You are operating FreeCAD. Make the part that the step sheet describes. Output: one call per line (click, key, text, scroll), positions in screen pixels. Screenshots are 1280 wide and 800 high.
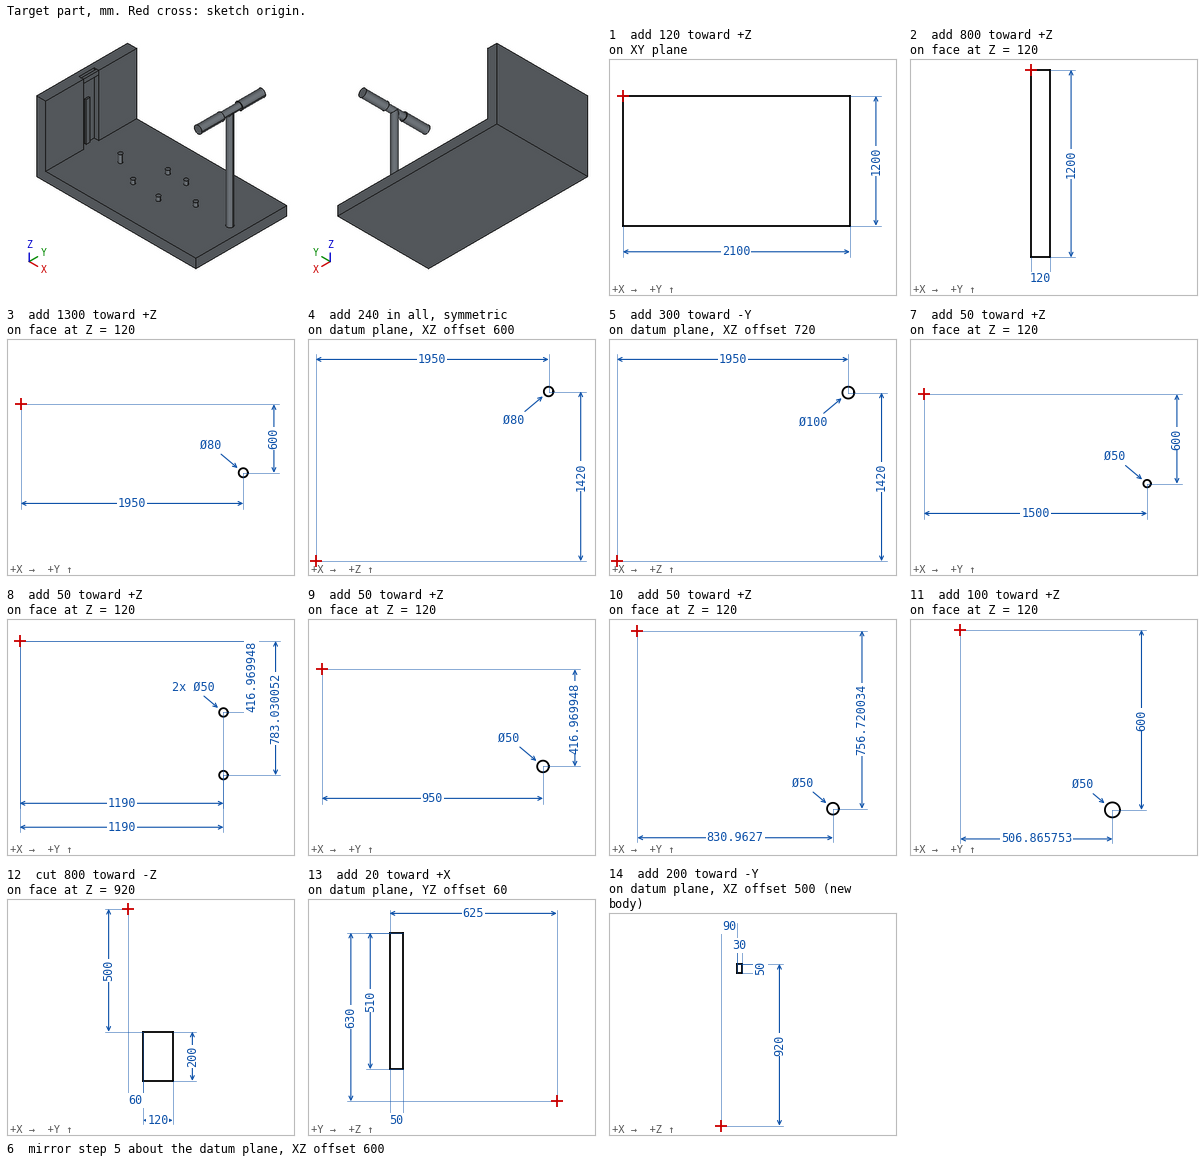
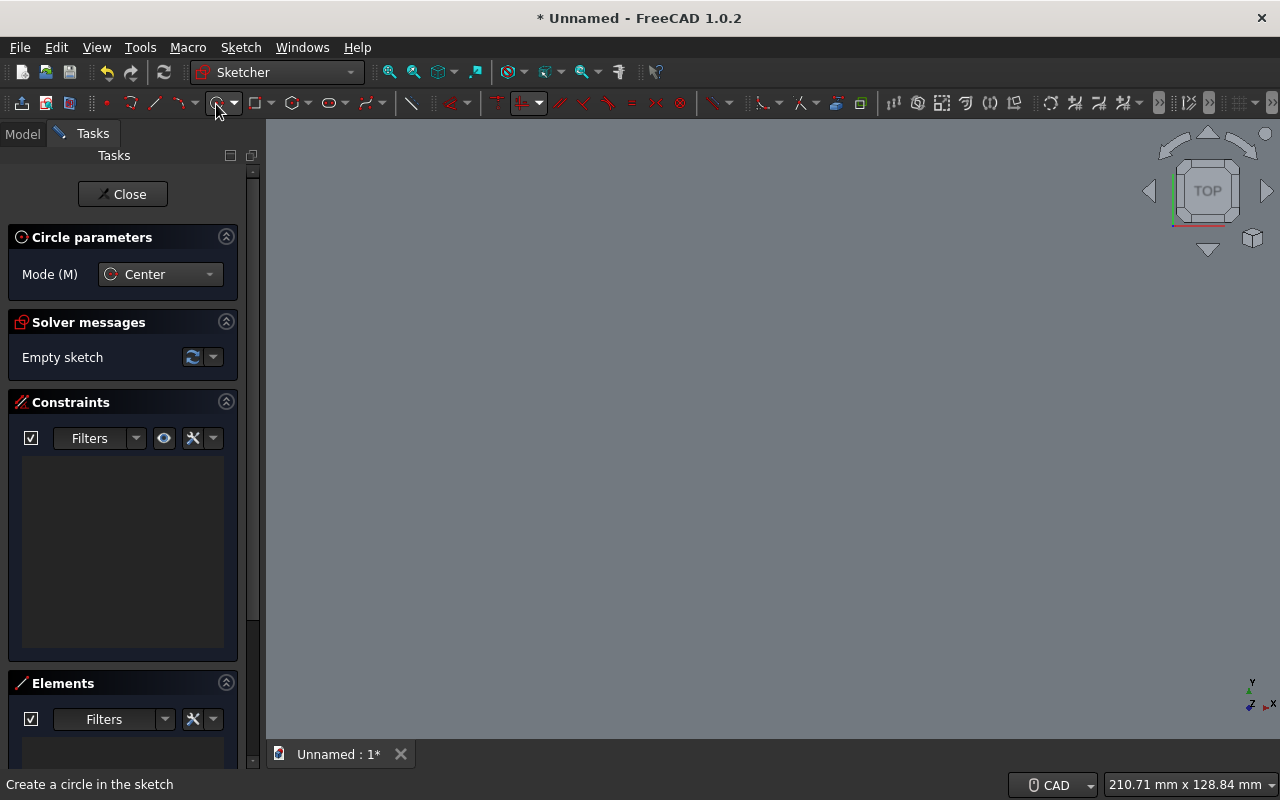
click(681, 419)
move(818, 283)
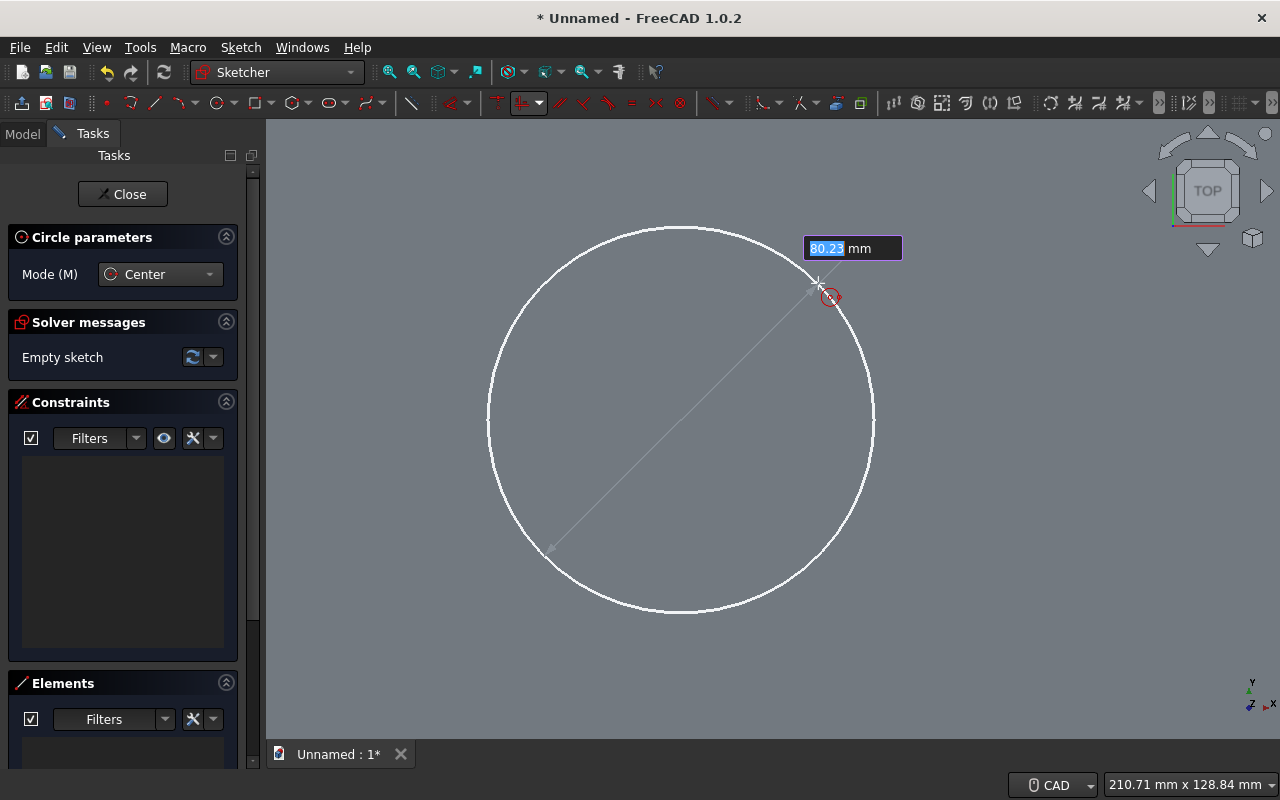
text(80)
key(Return)
key(Escape)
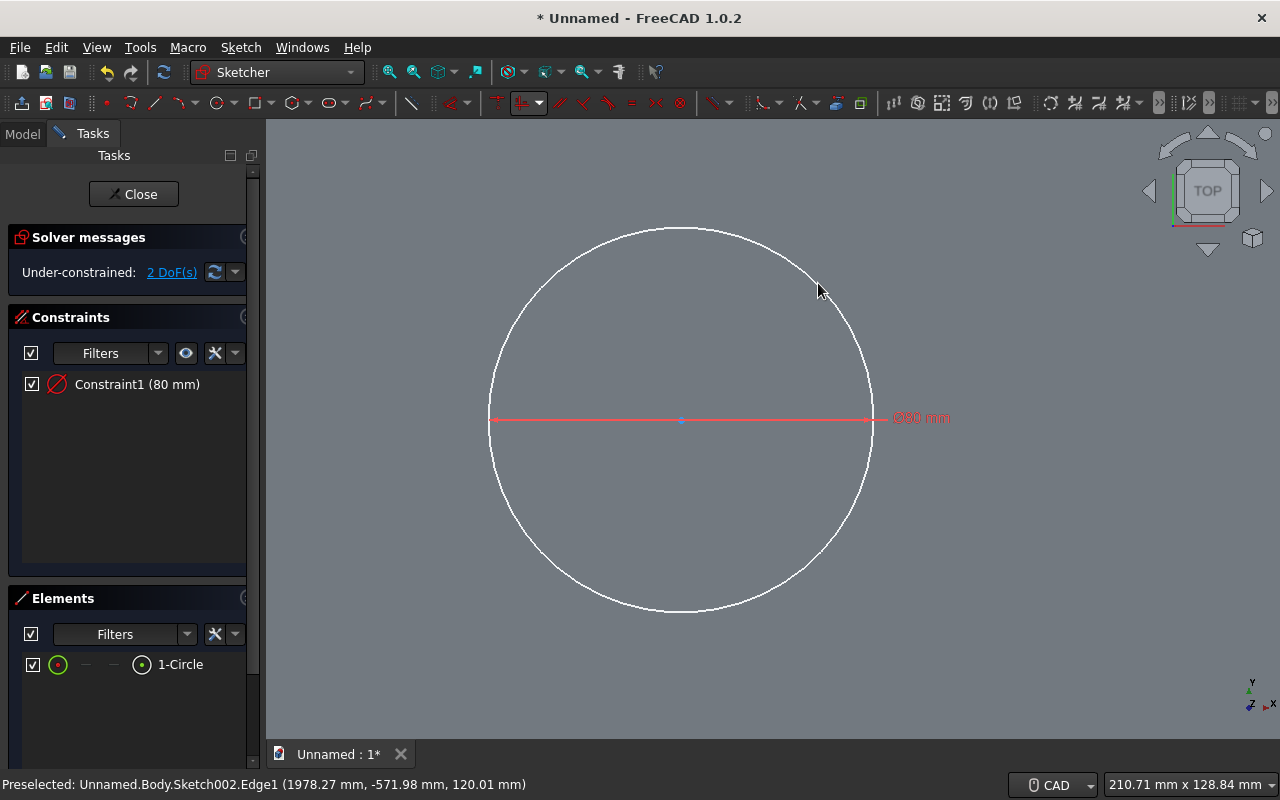
click(450, 104)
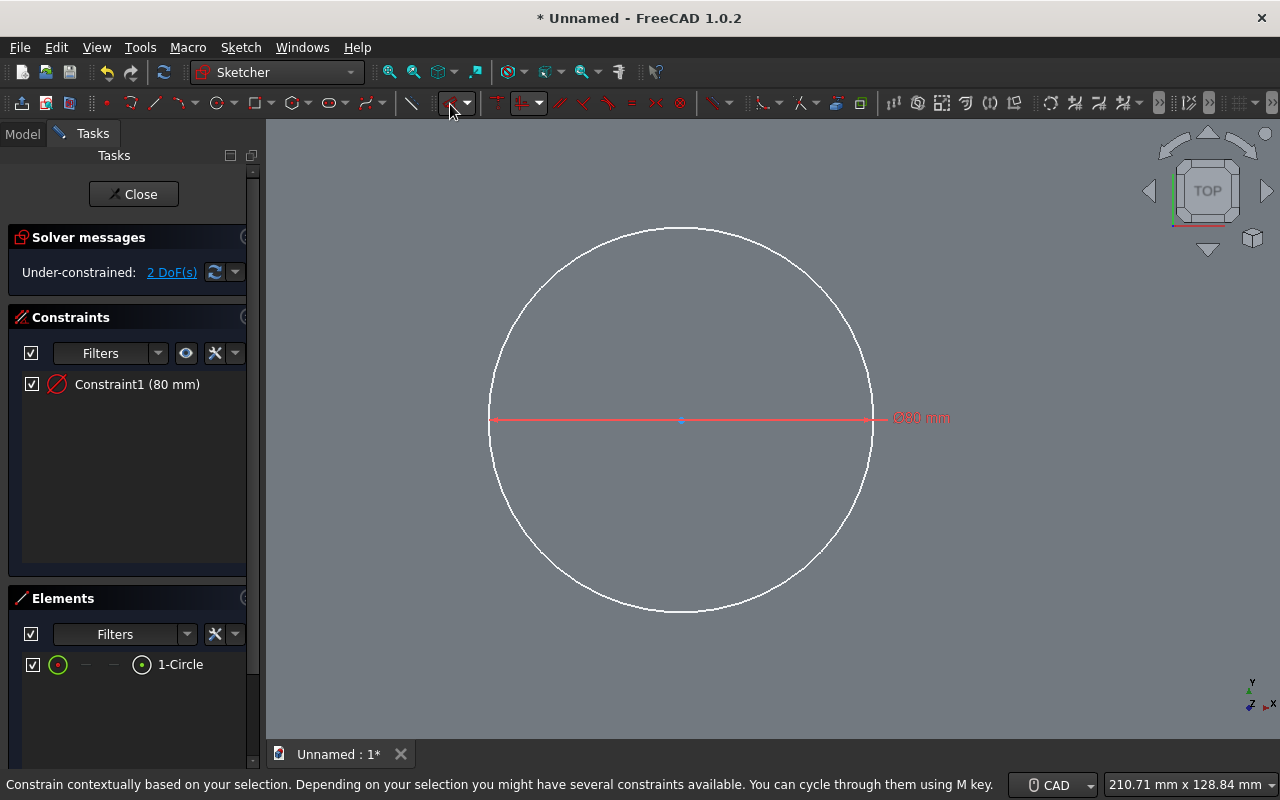
click(681, 420)
click(715, 284)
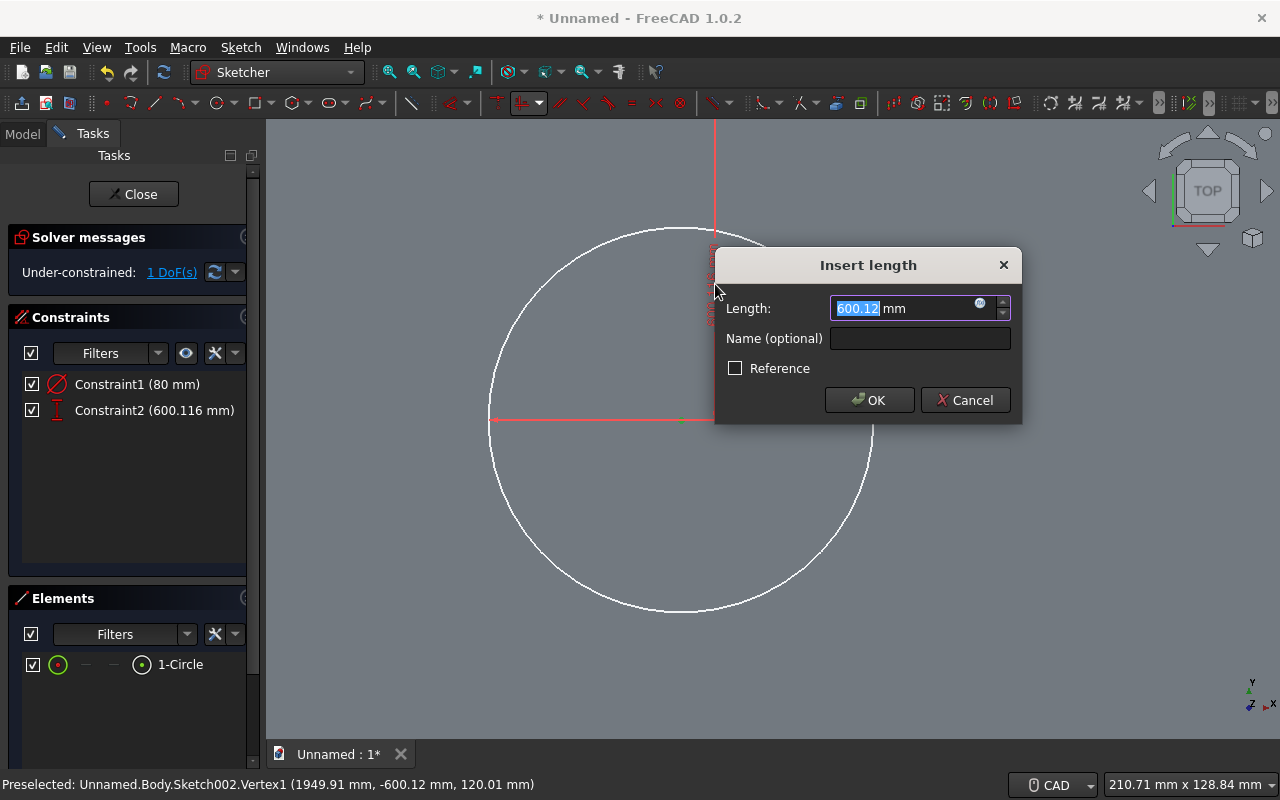
text(600)
key(Return)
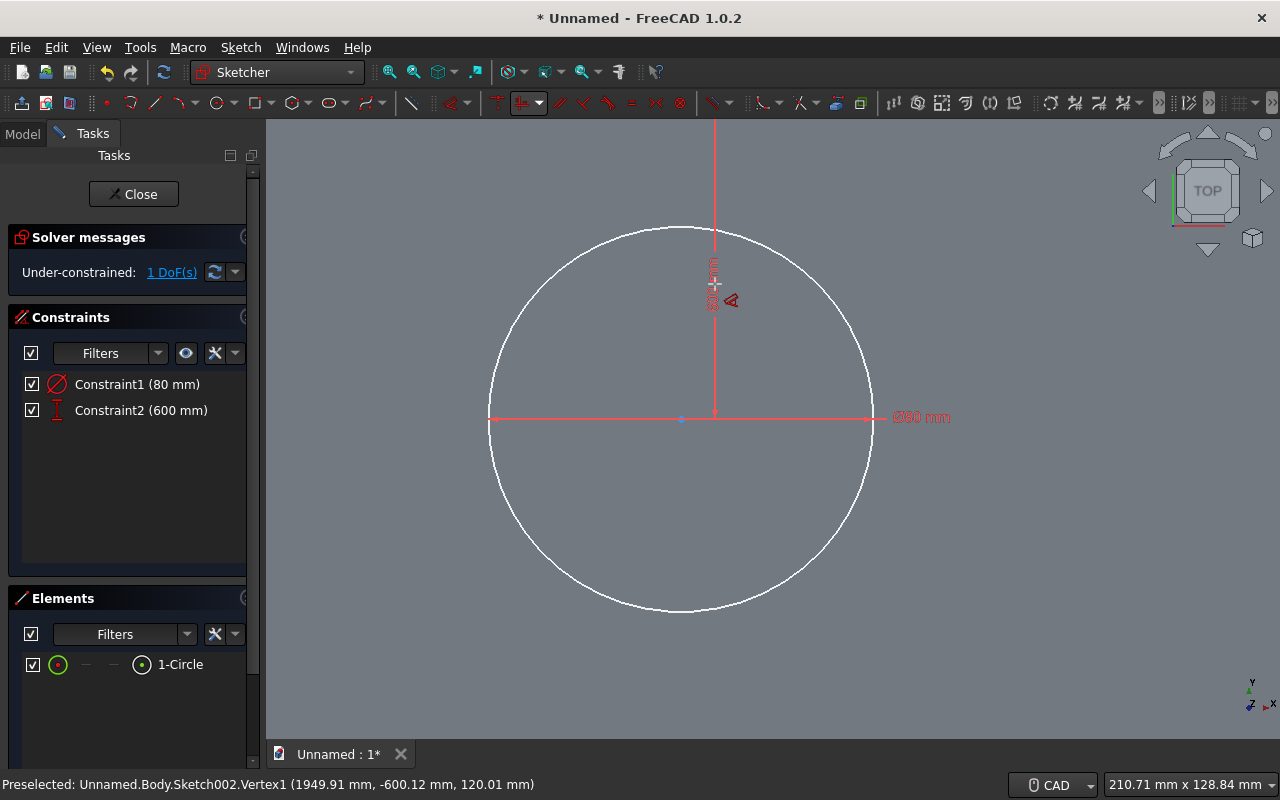
click(681, 419)
click(398, 453)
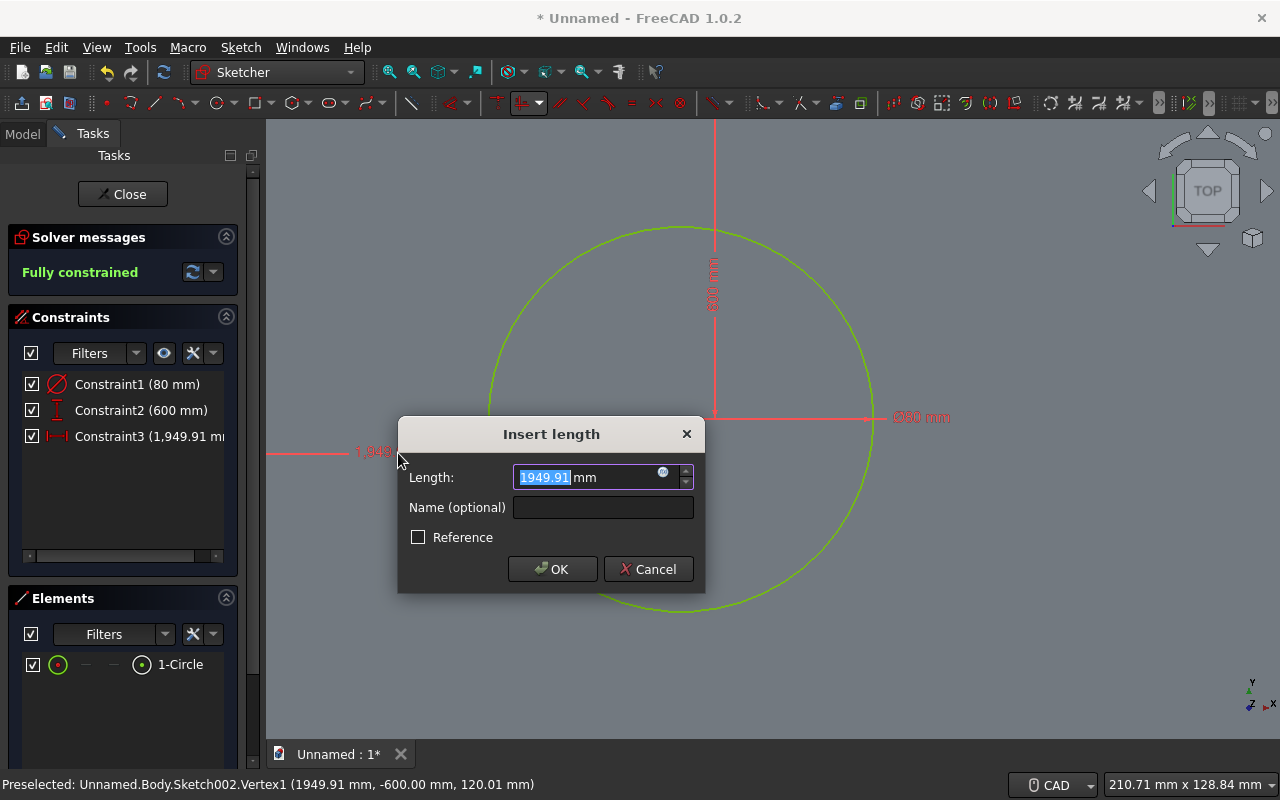
text(1950)
key(Return)
key(Escape)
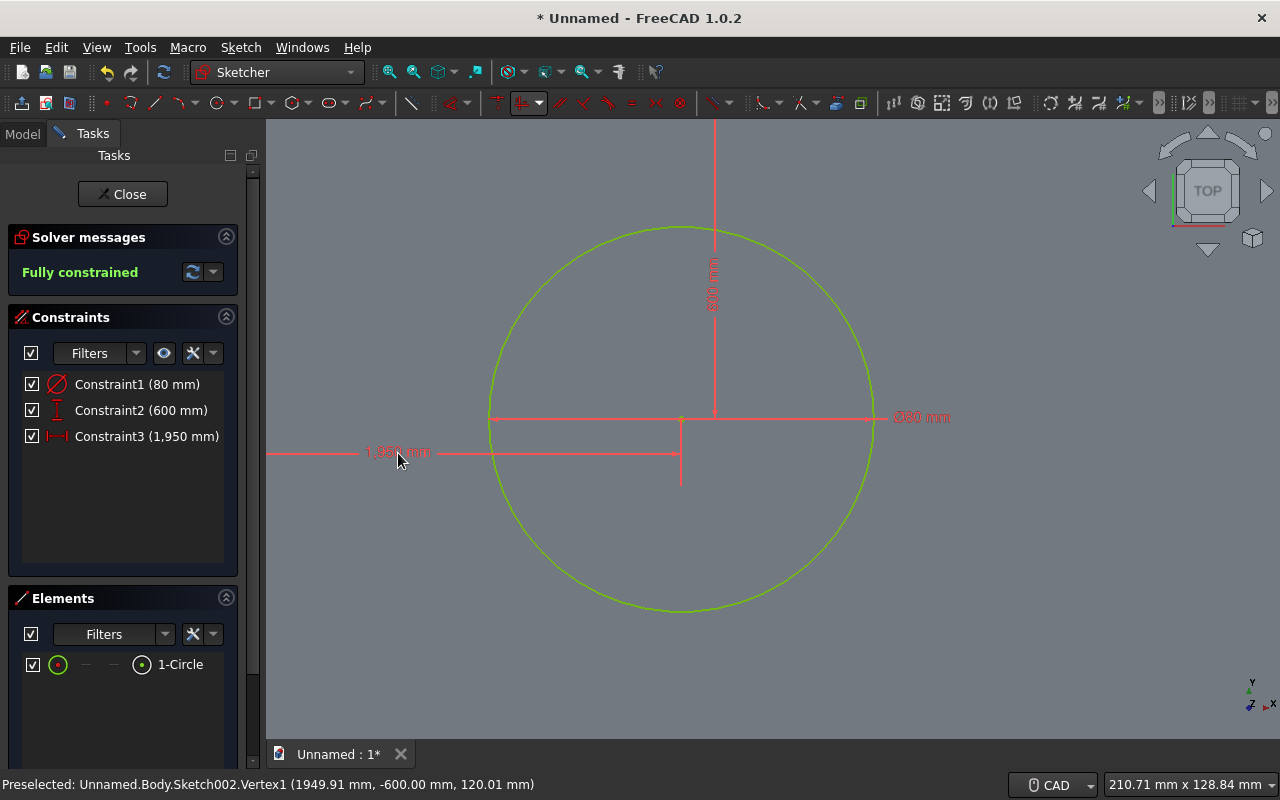
click(123, 194)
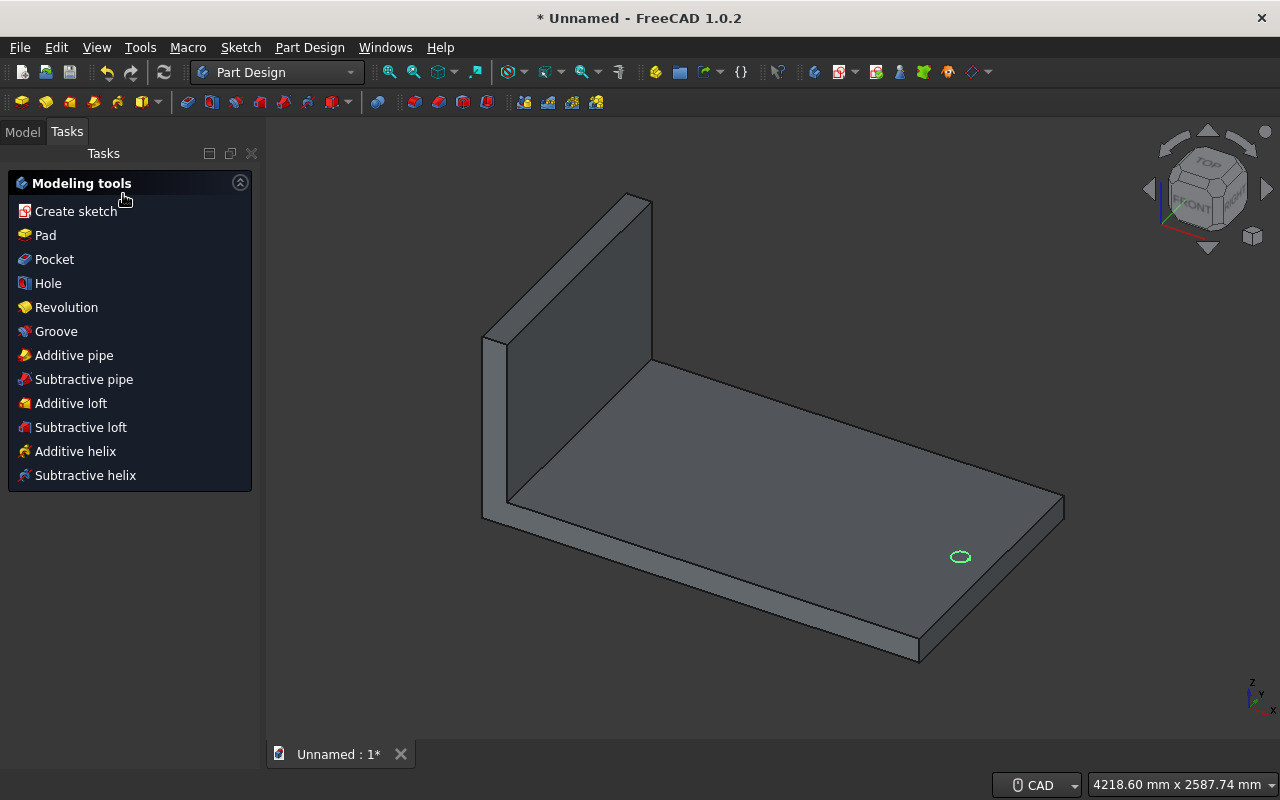
click(22, 102)